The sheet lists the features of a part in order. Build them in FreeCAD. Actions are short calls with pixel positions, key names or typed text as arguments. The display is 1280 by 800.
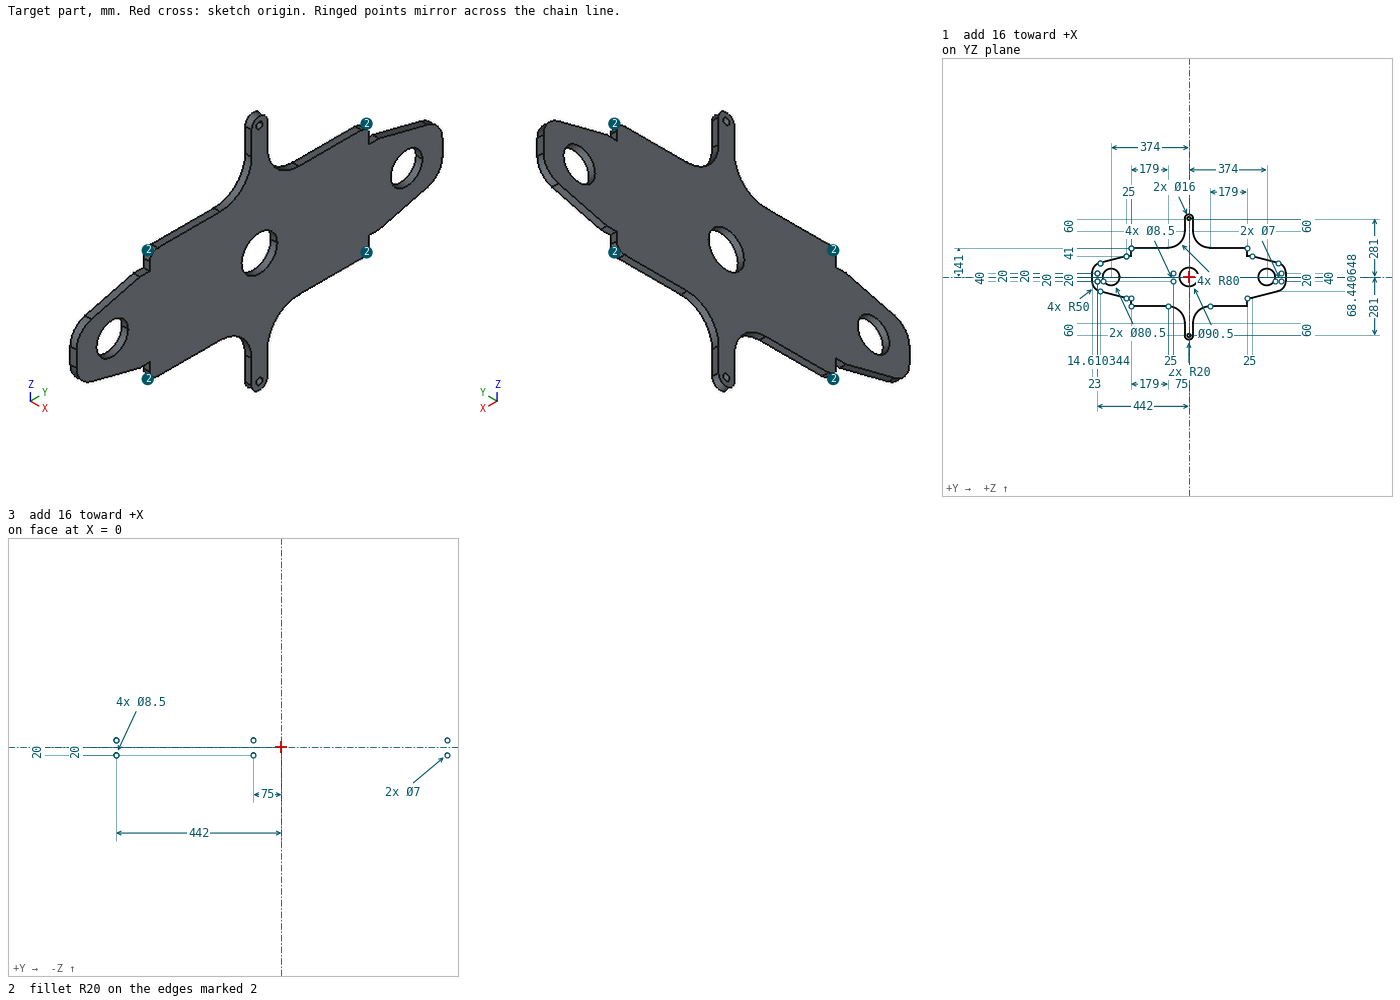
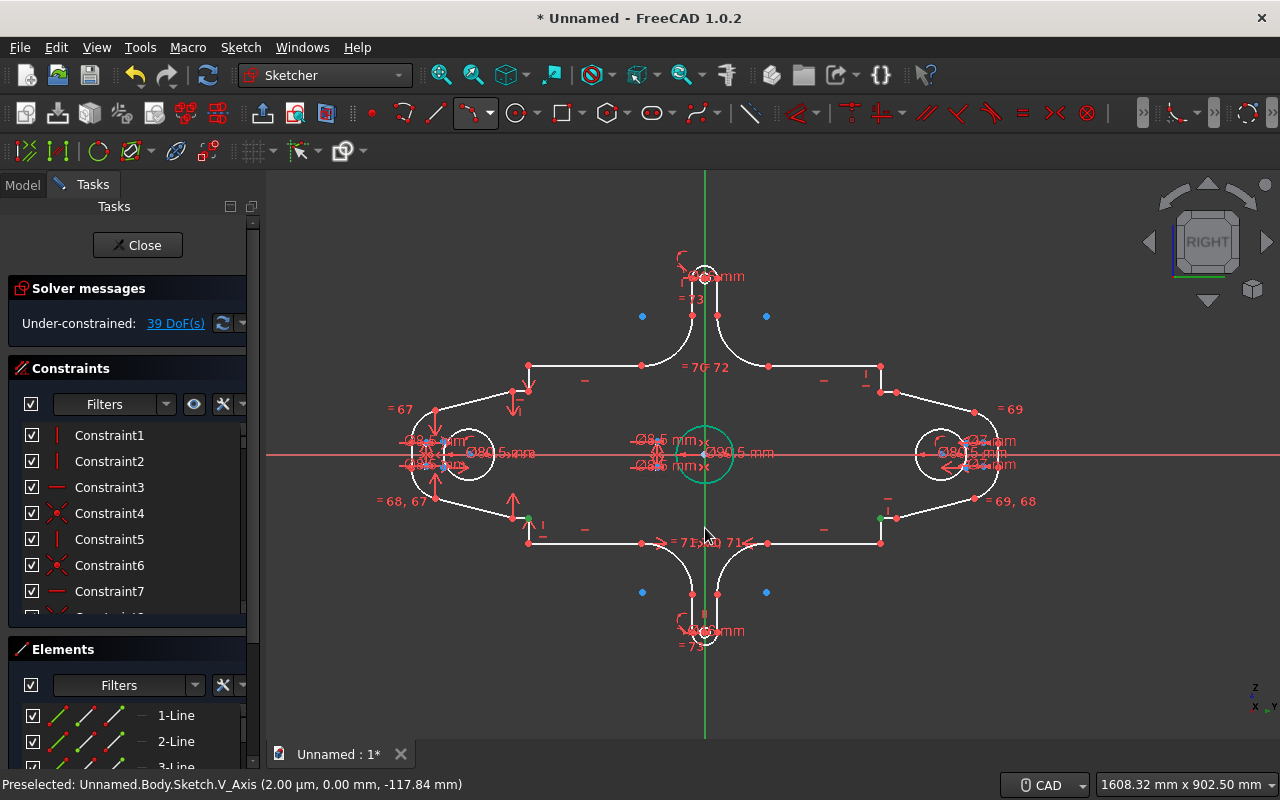
click(1056, 114)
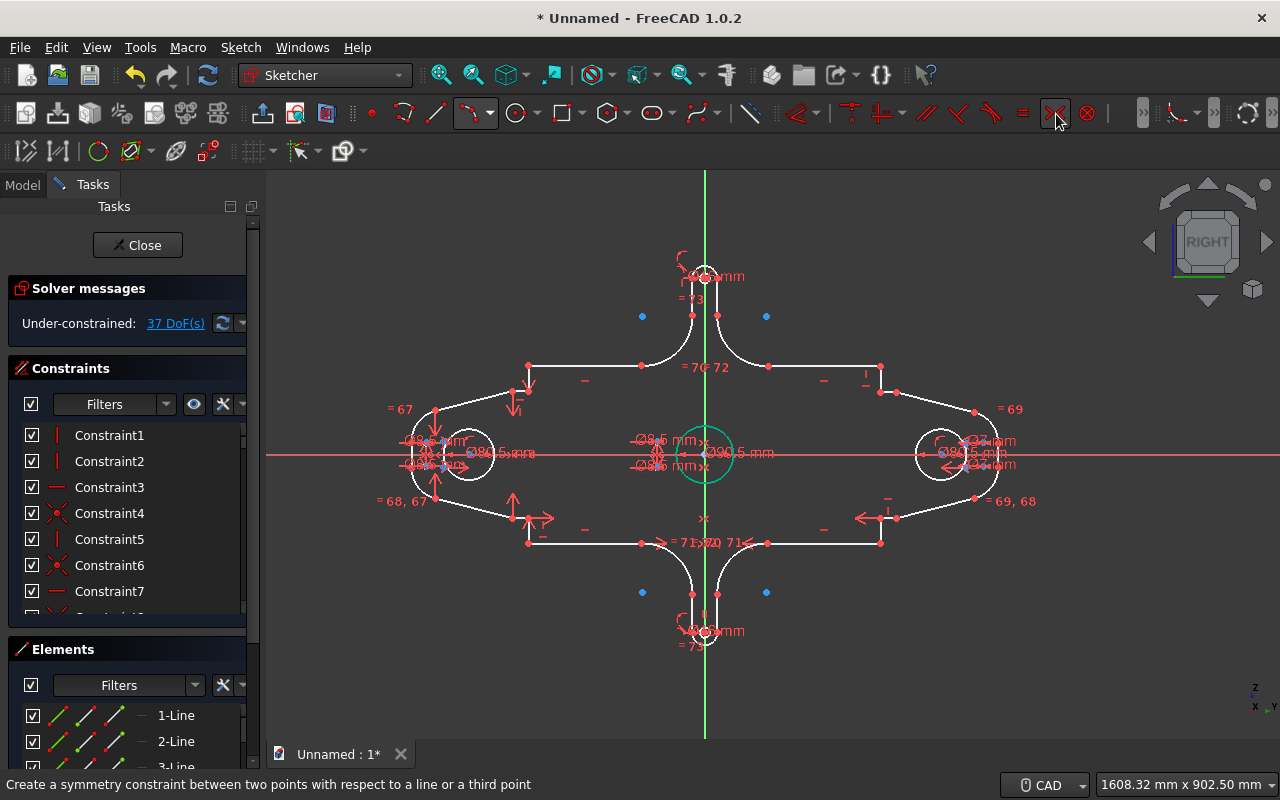
click(435, 411)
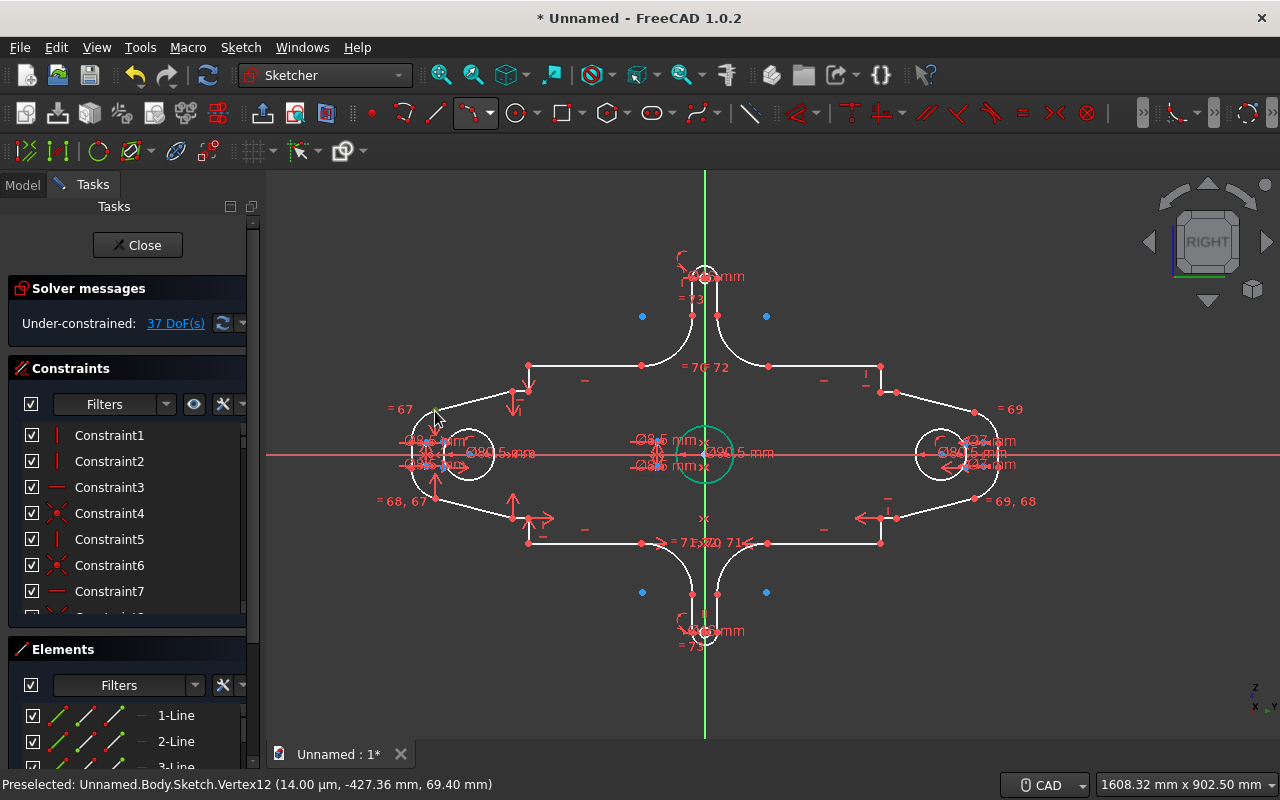
click(974, 412)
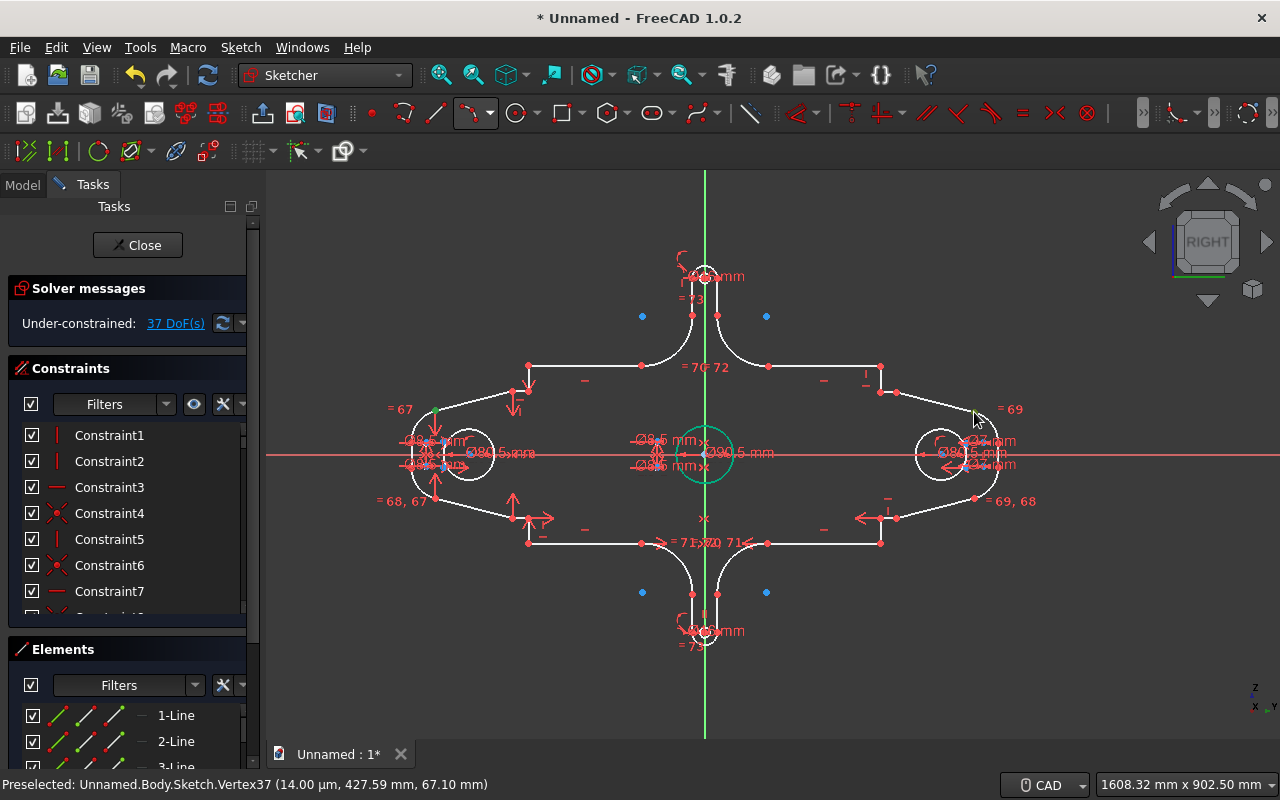
click(705, 528)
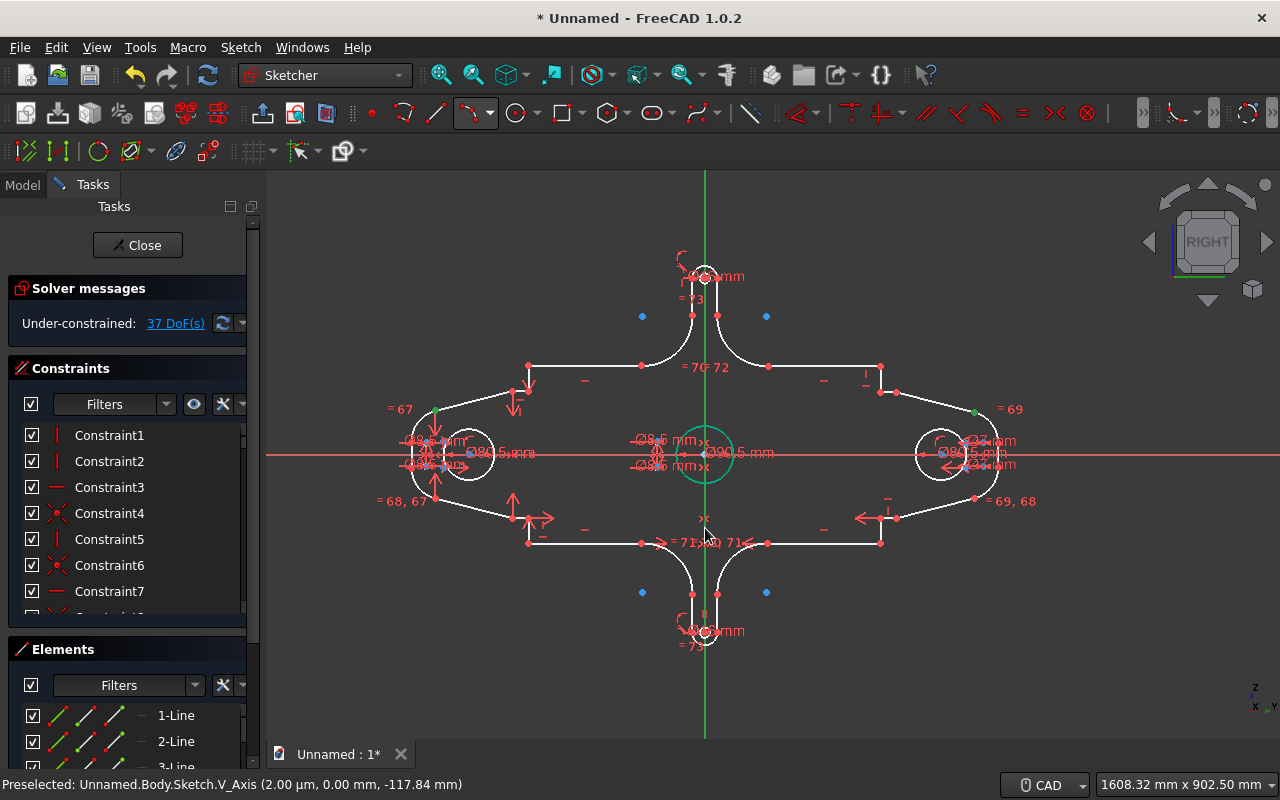
click(1056, 114)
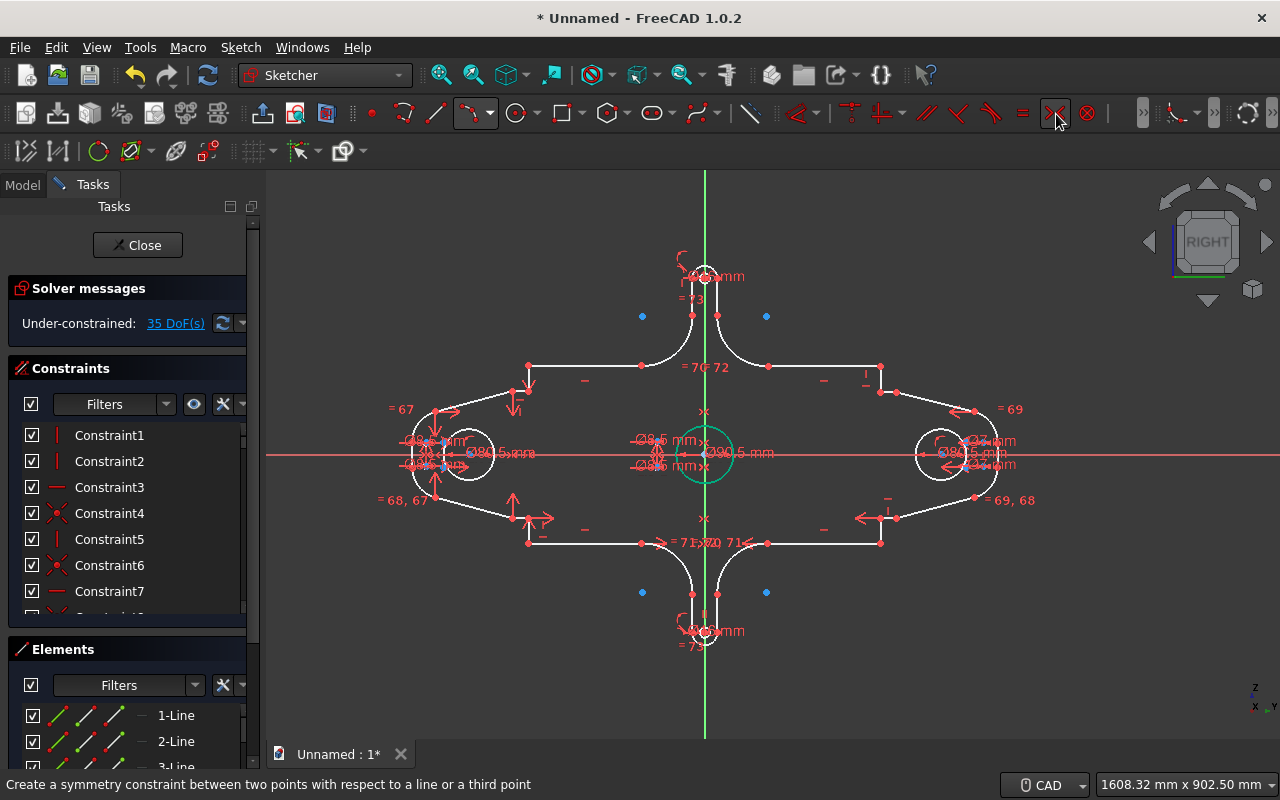
click(513, 391)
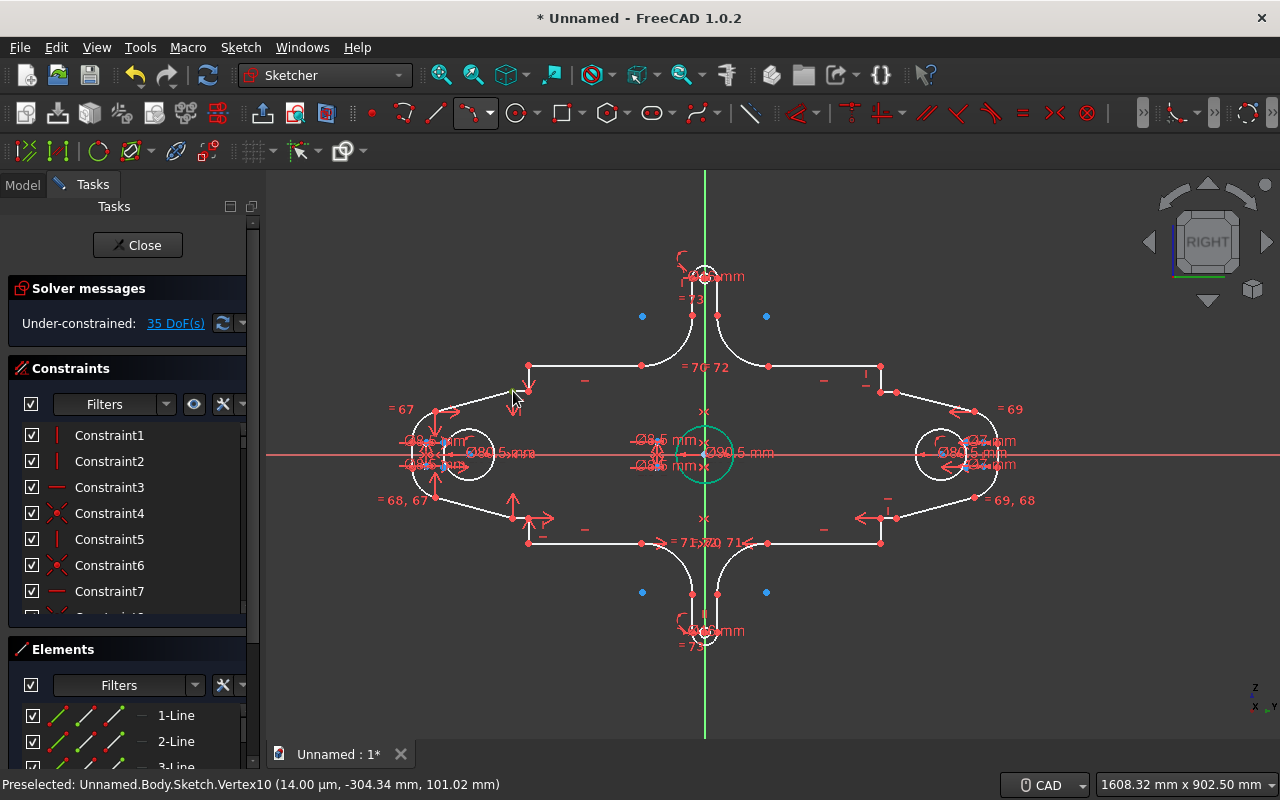
click(896, 392)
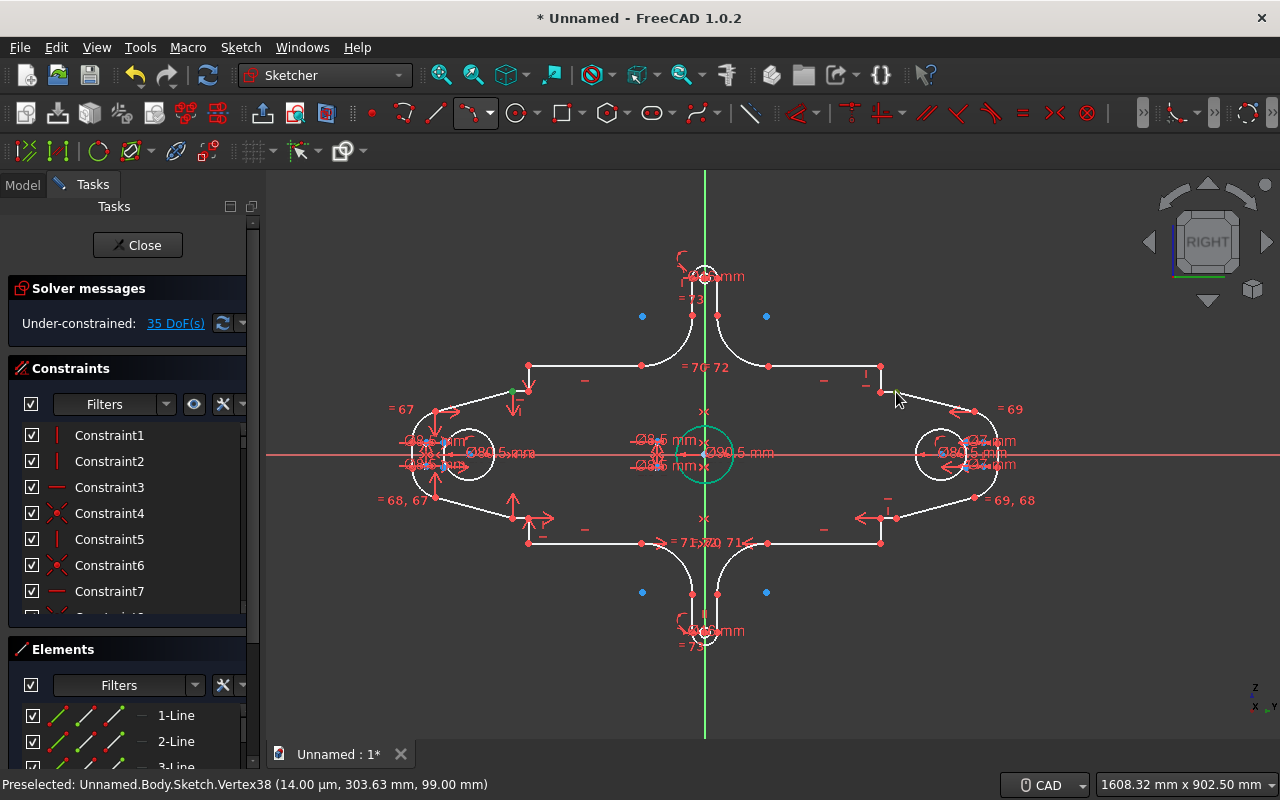
click(705, 528)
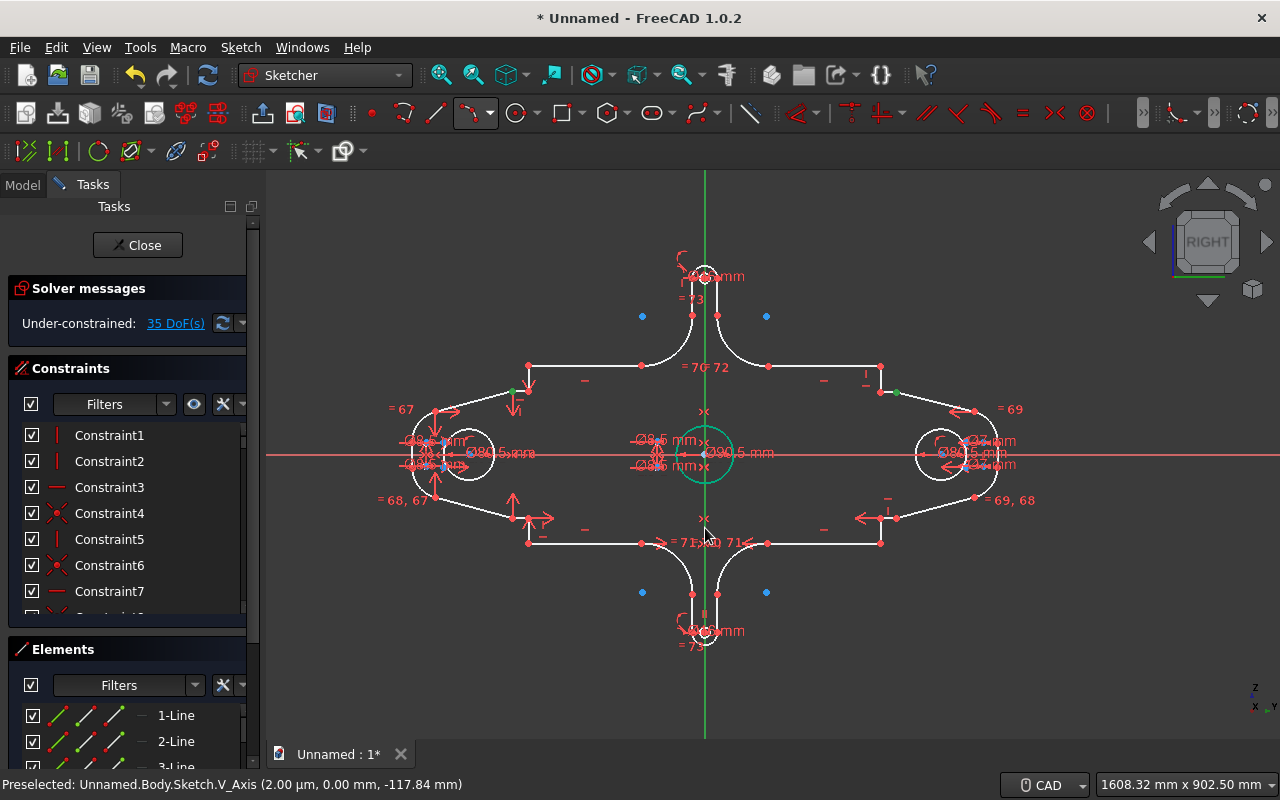
click(1056, 114)